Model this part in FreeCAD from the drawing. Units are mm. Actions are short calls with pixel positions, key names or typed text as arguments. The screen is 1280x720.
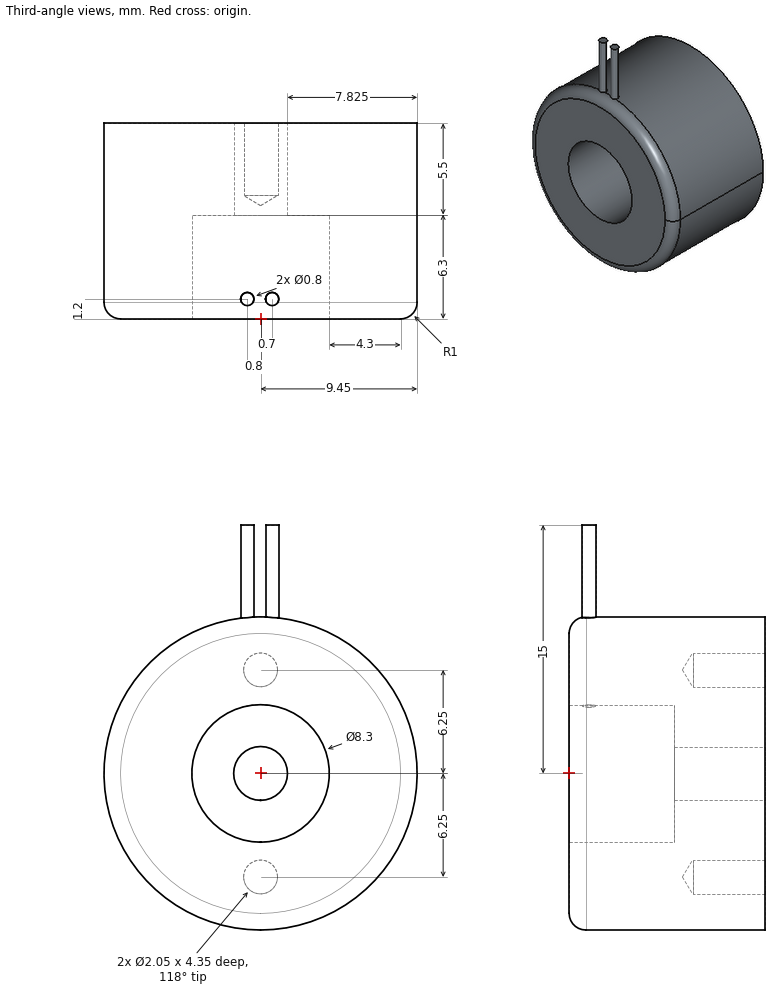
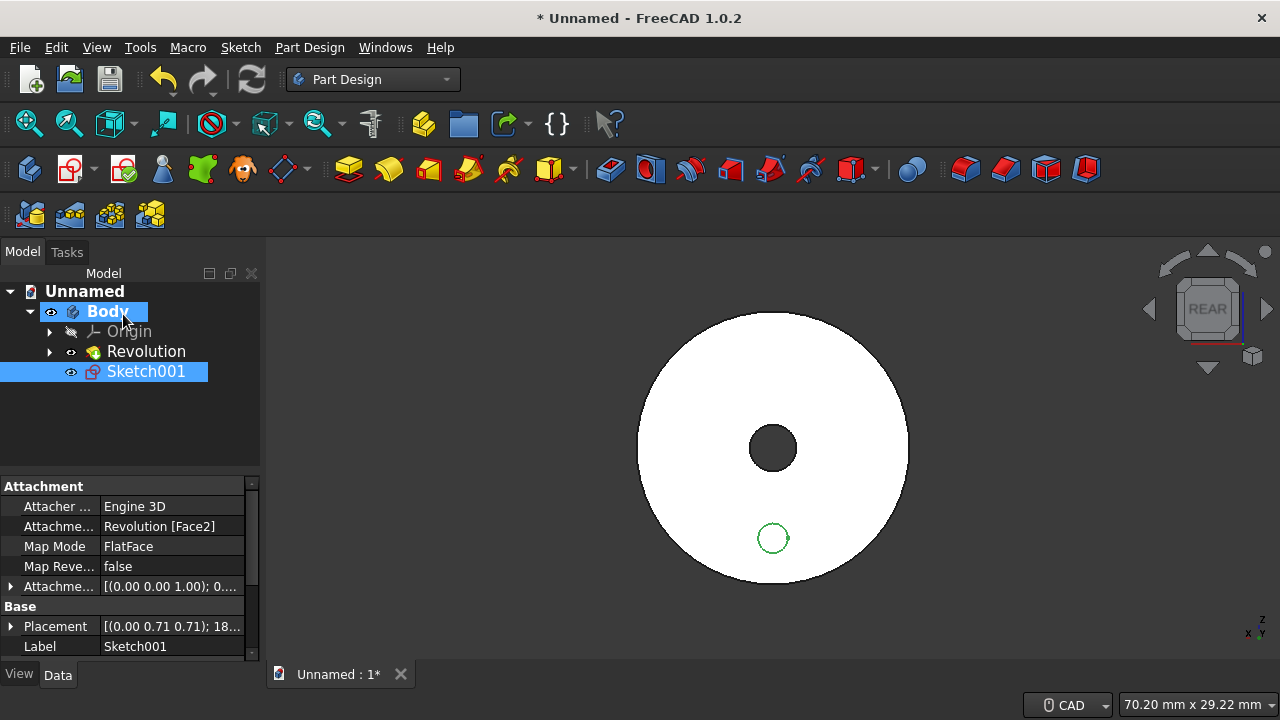
click(652, 170)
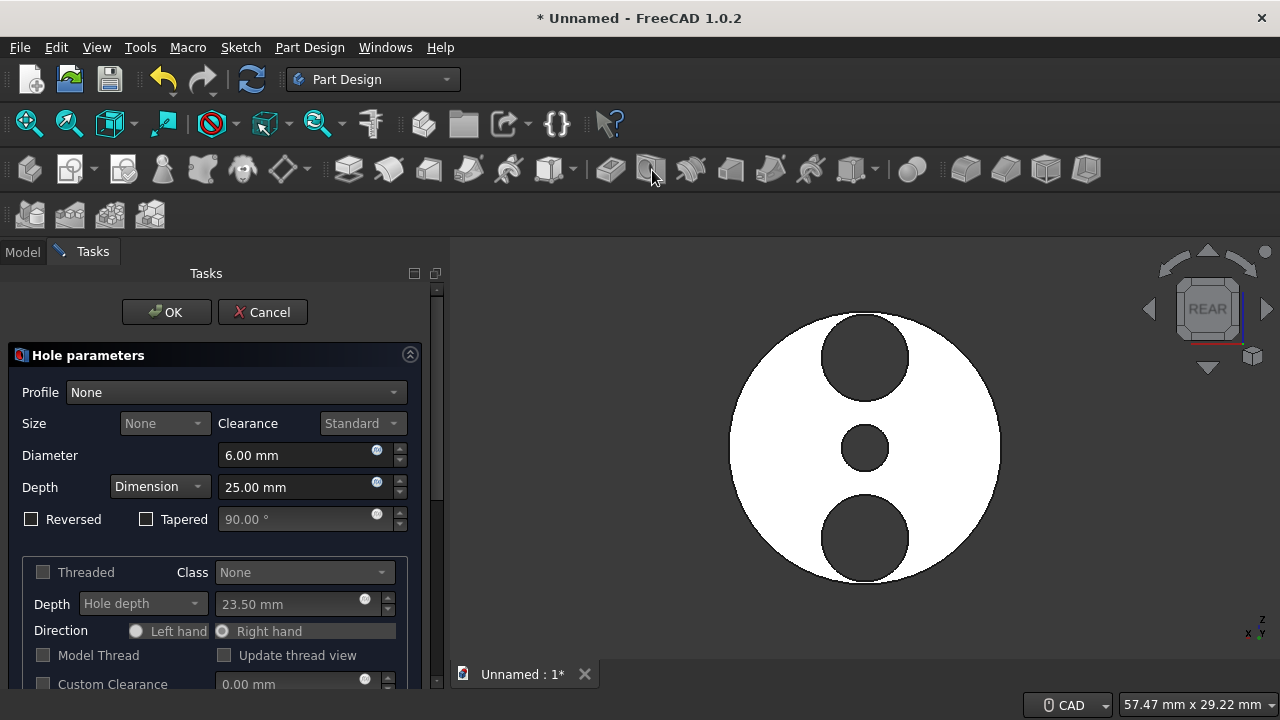
triple_click(305, 455)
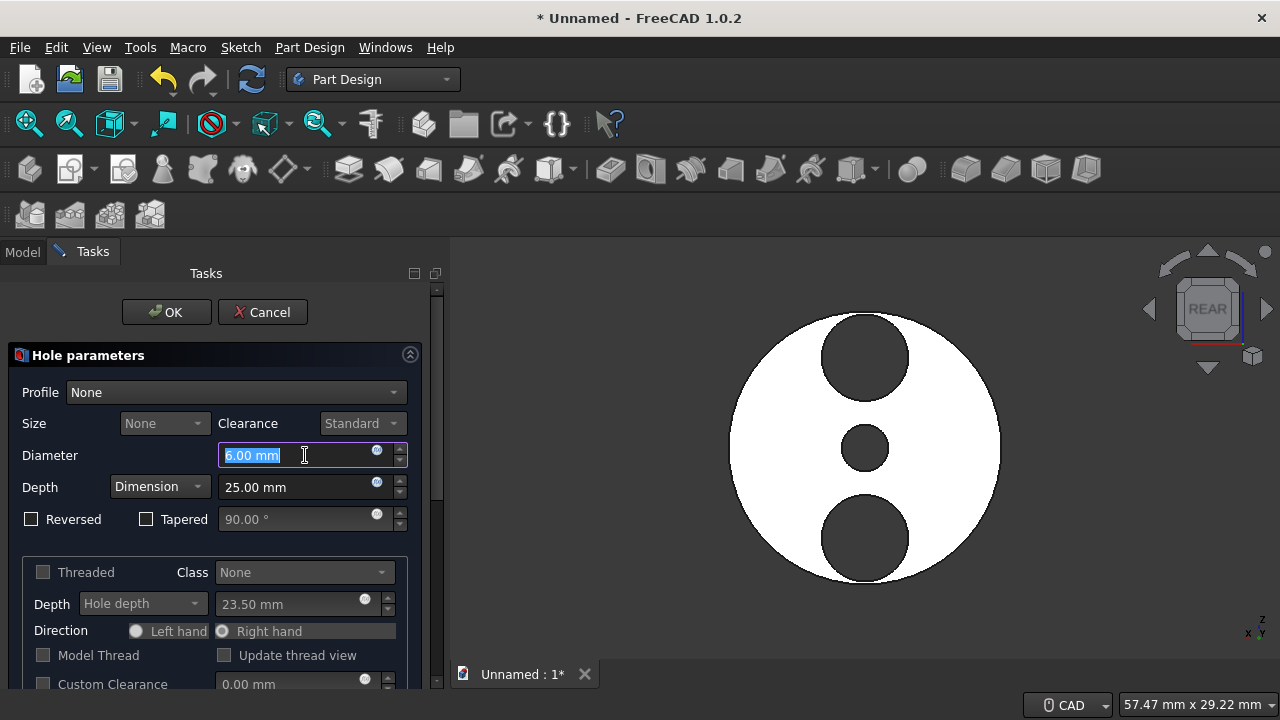
text(2.05)
key(Tab)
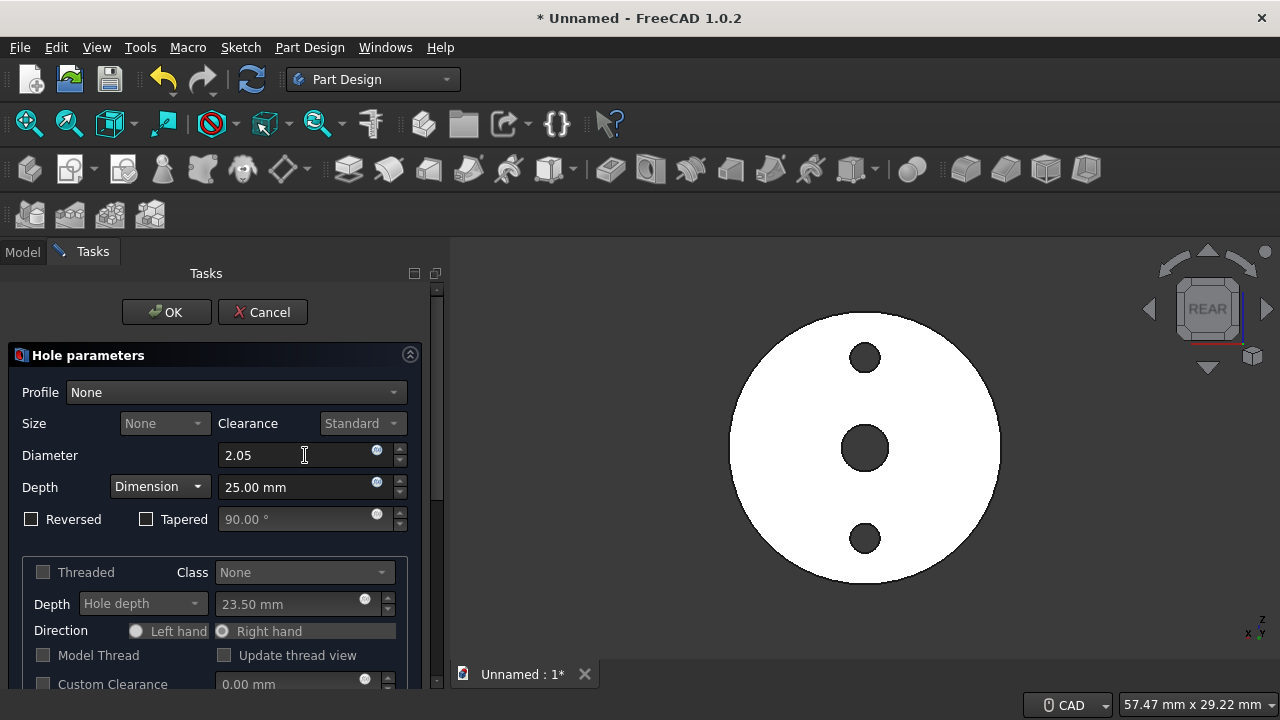
triple_click(305, 487)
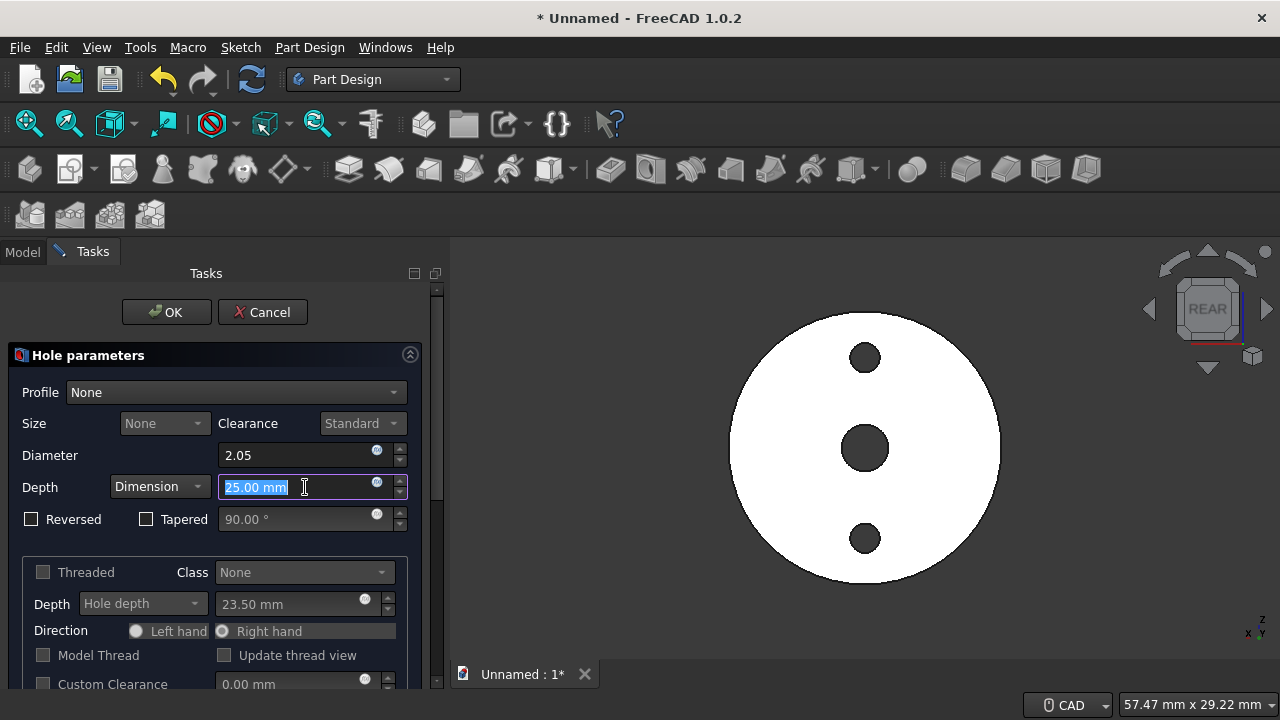
text(4.35)
key(Tab)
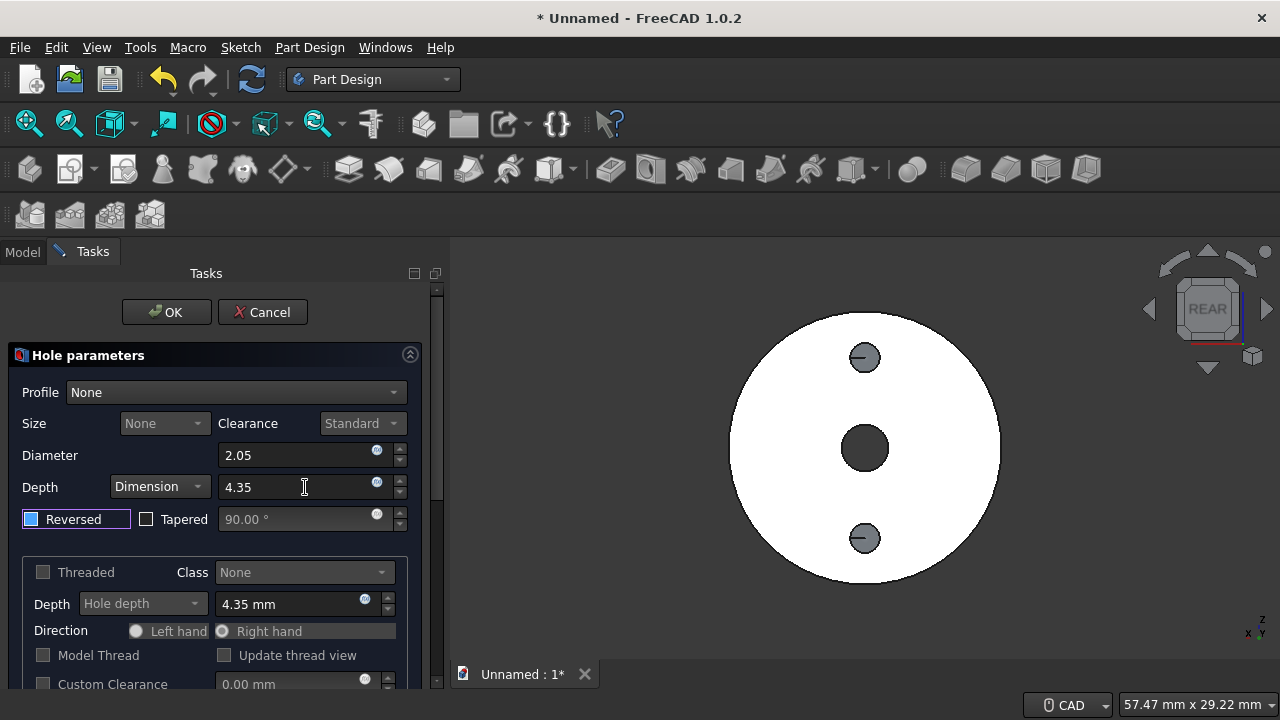
click(167, 312)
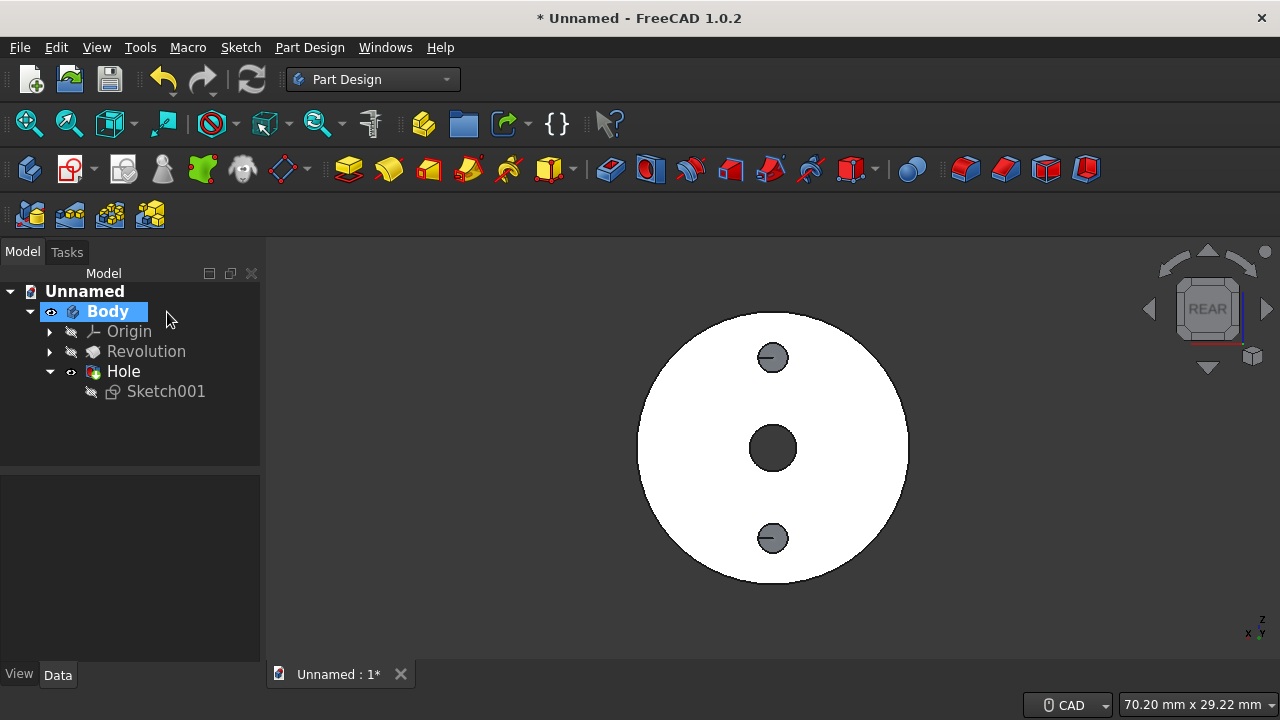
click(70, 170)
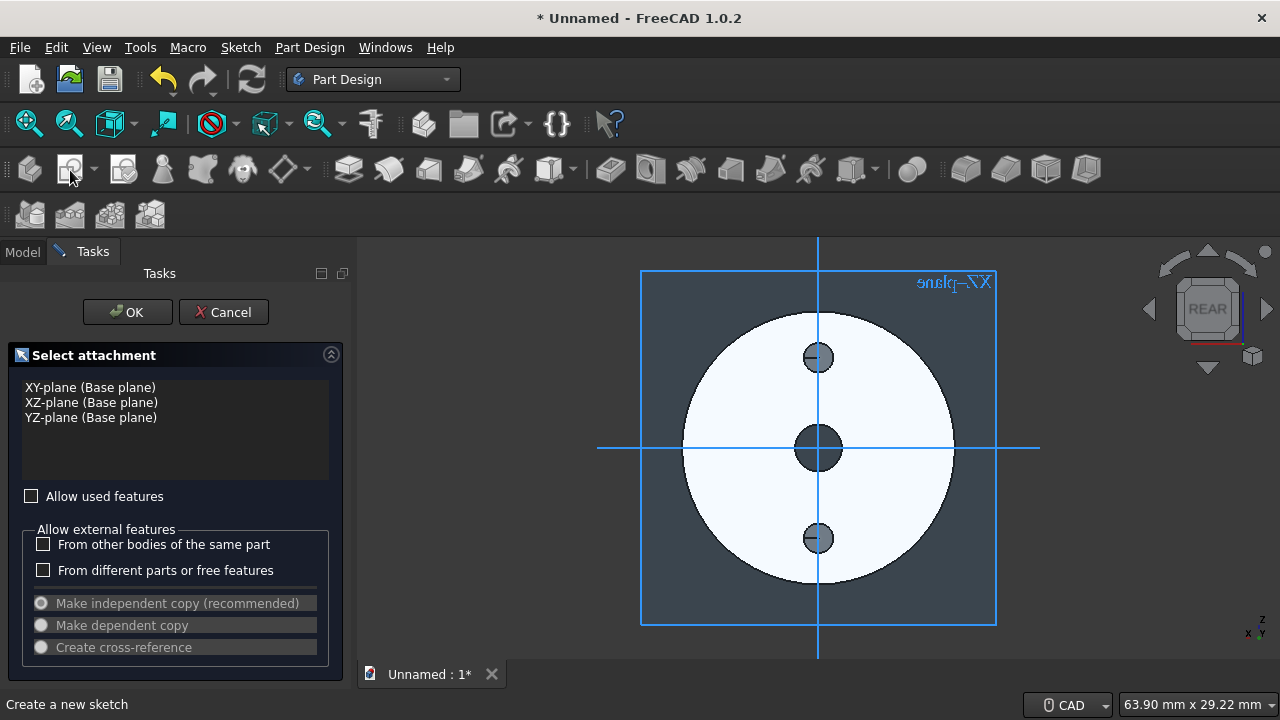
click(82, 388)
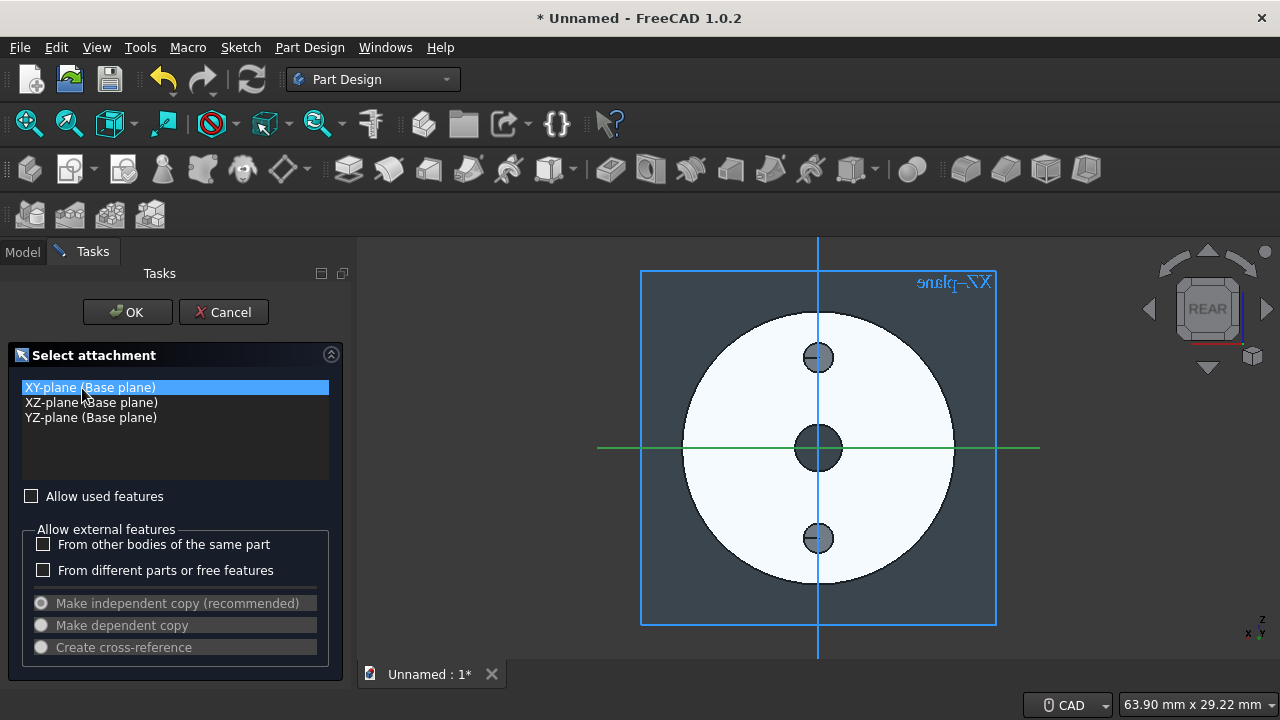
click(128, 312)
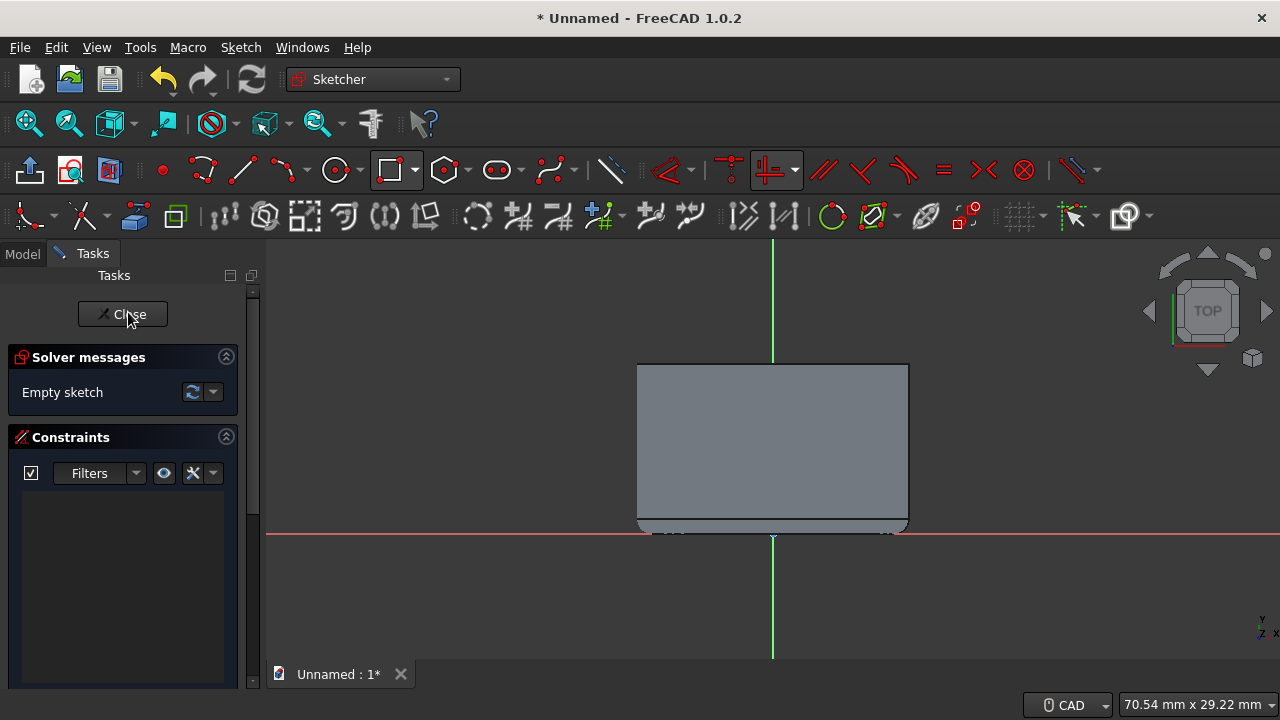
click(110, 170)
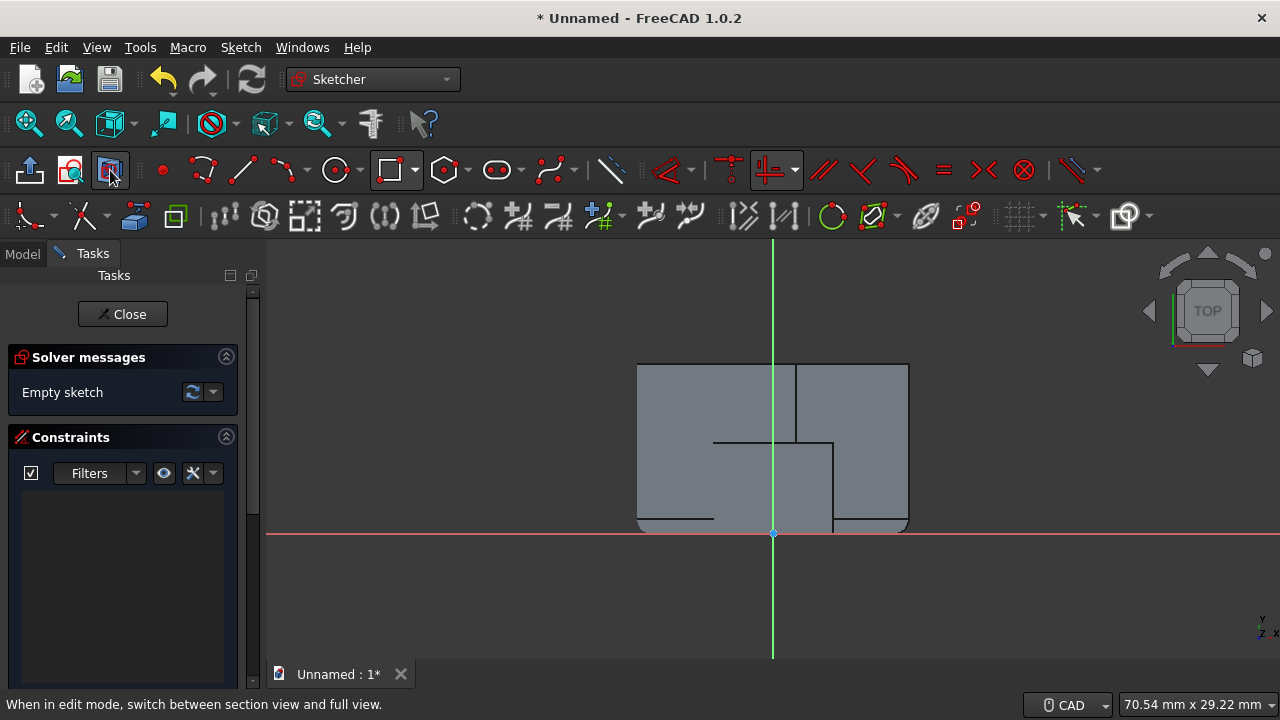
scroll(779, 530, up, 12)